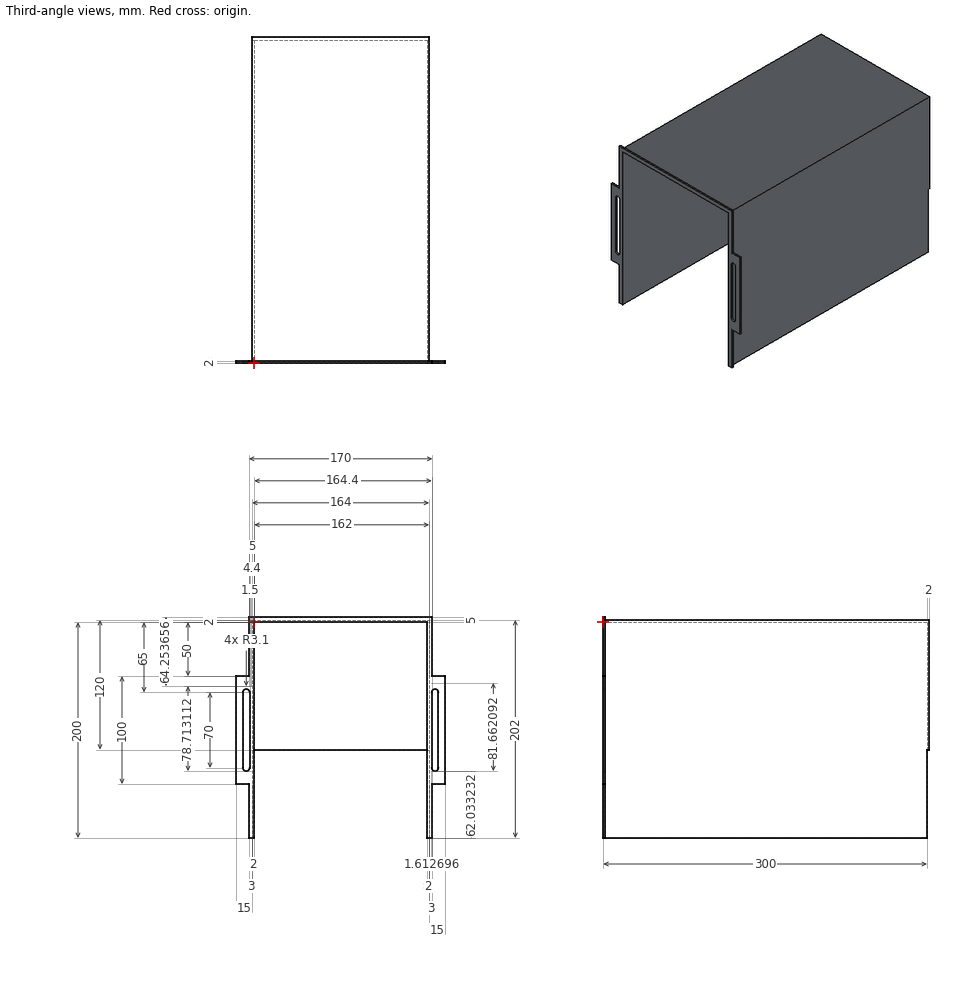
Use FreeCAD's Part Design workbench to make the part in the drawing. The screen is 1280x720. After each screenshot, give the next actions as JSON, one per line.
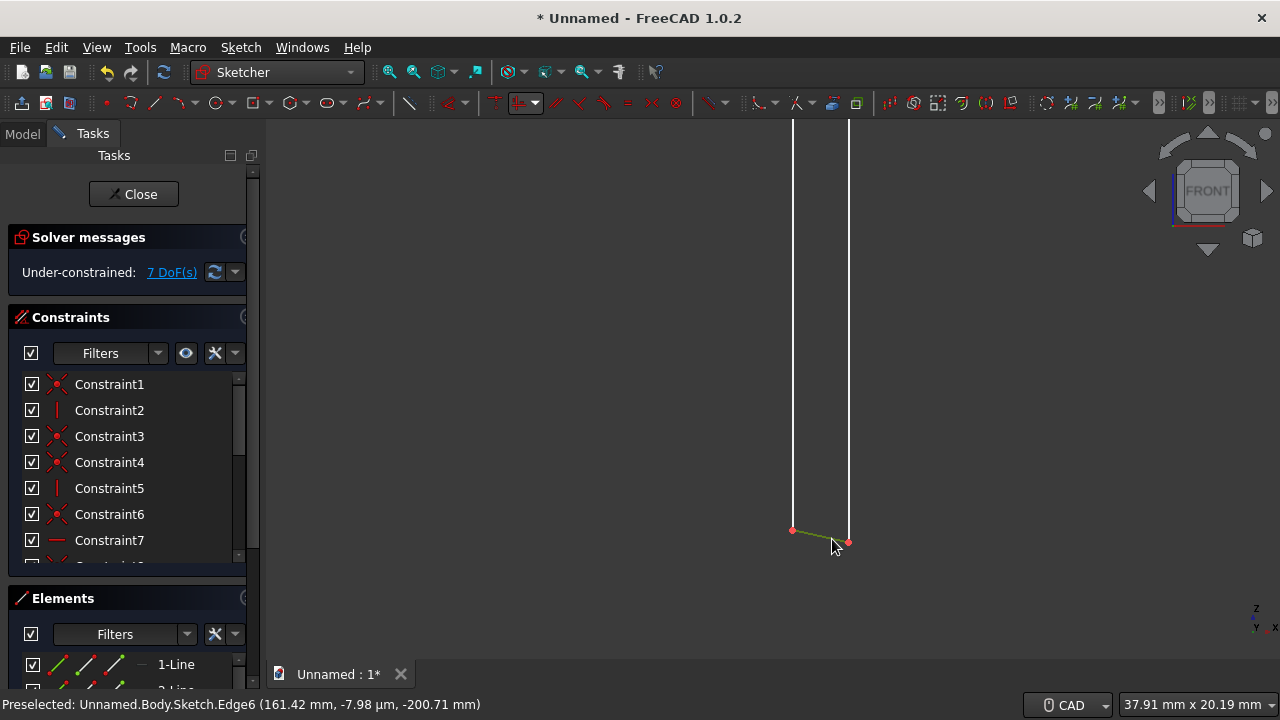
{"action": "key", "text": "h"}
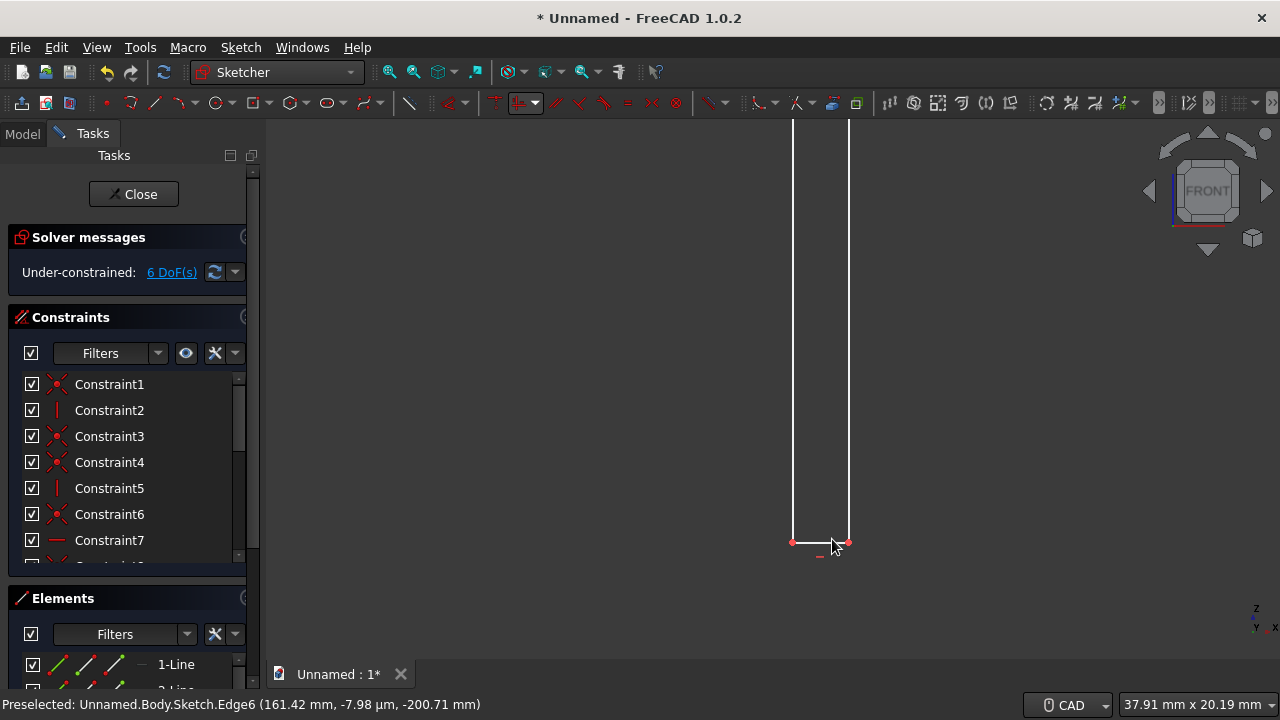
{"action": "left_click", "coordinate": [448, 104]}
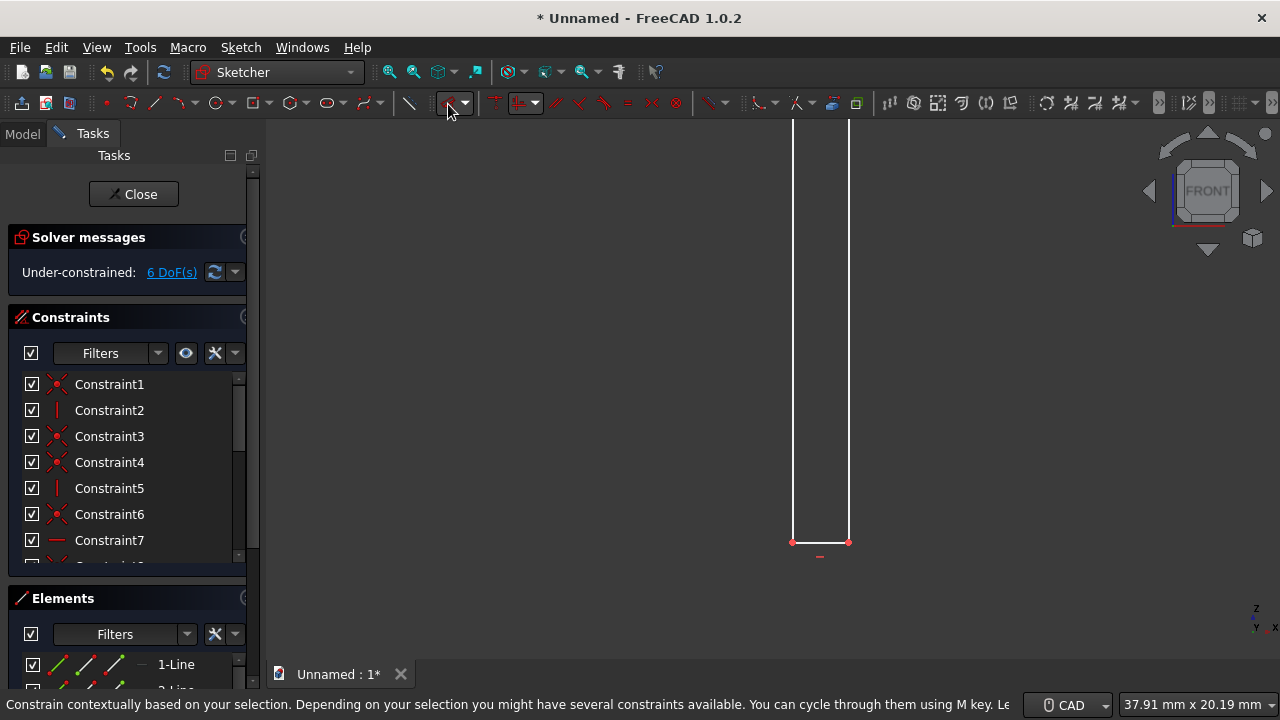
{"action": "scroll", "coordinate": [837, 555], "scroll_direction": "down", "scroll_amount": 14}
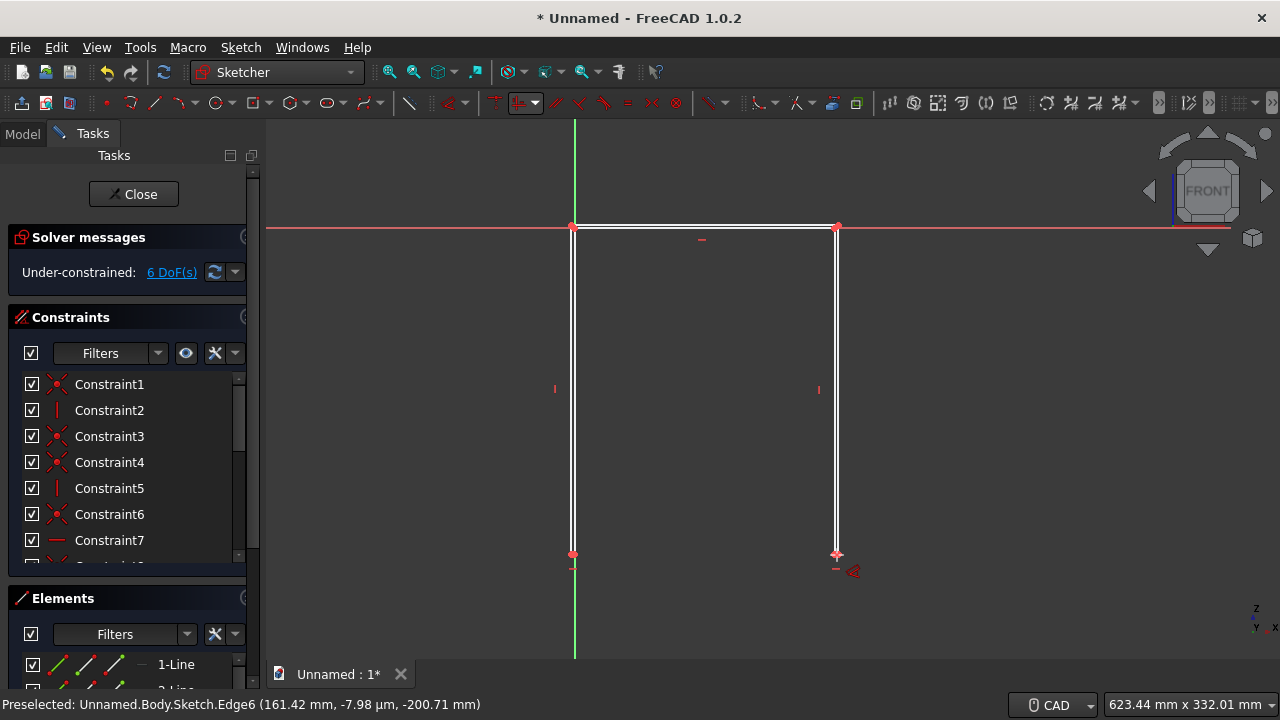
{"action": "scroll", "coordinate": [574, 555], "scroll_direction": "up", "scroll_amount": 14}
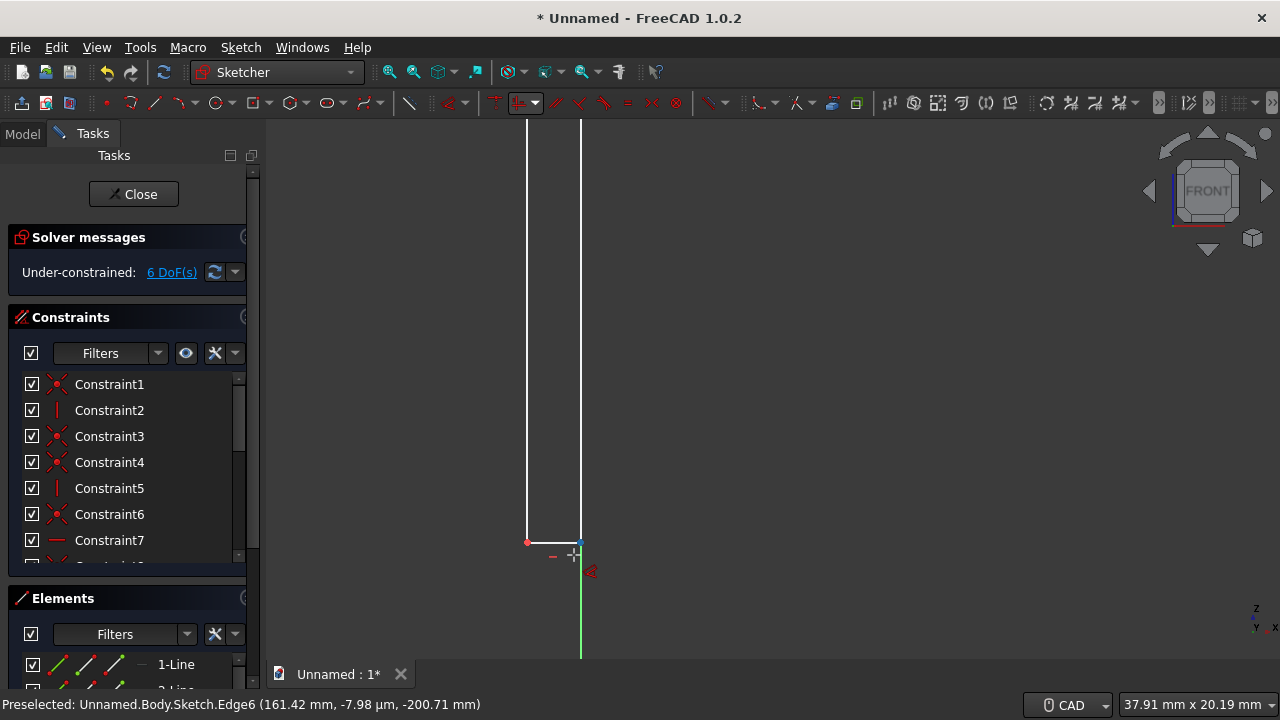
{"action": "left_click", "coordinate": [565, 543]}
{"action": "left_click", "coordinate": [554, 577]}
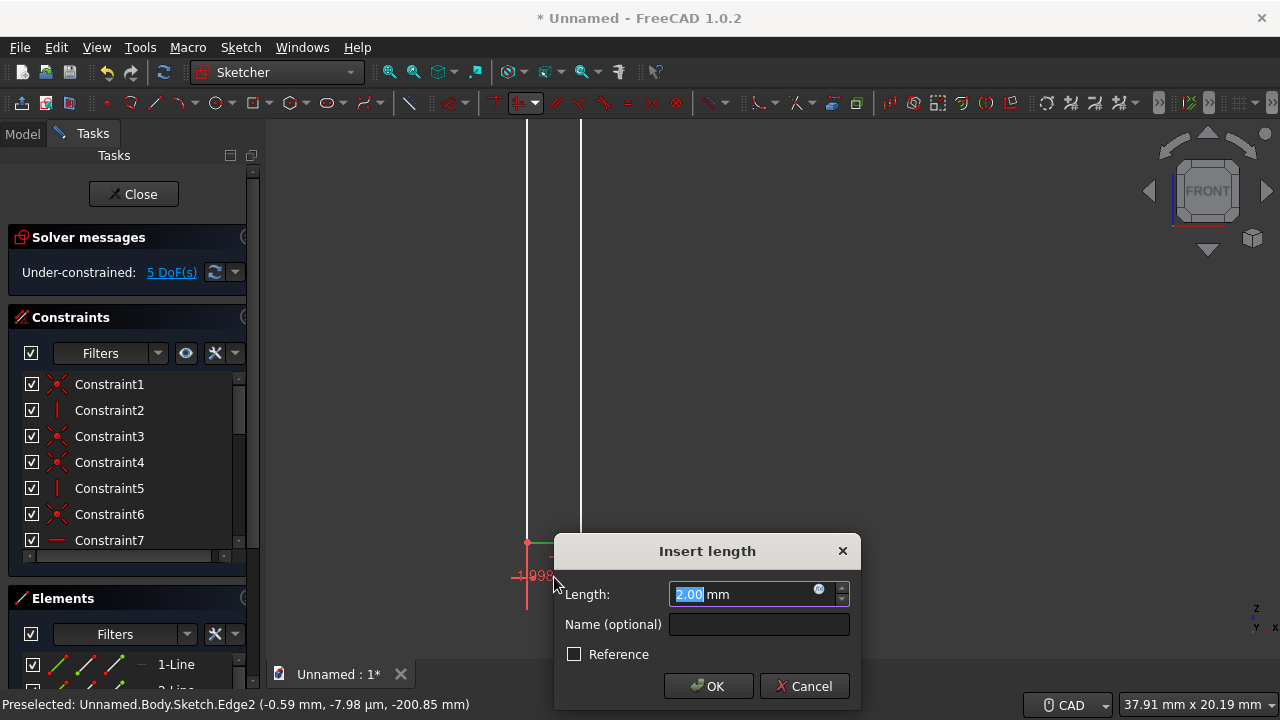
{"action": "type", "text": "2"}
{"action": "key", "text": "Return"}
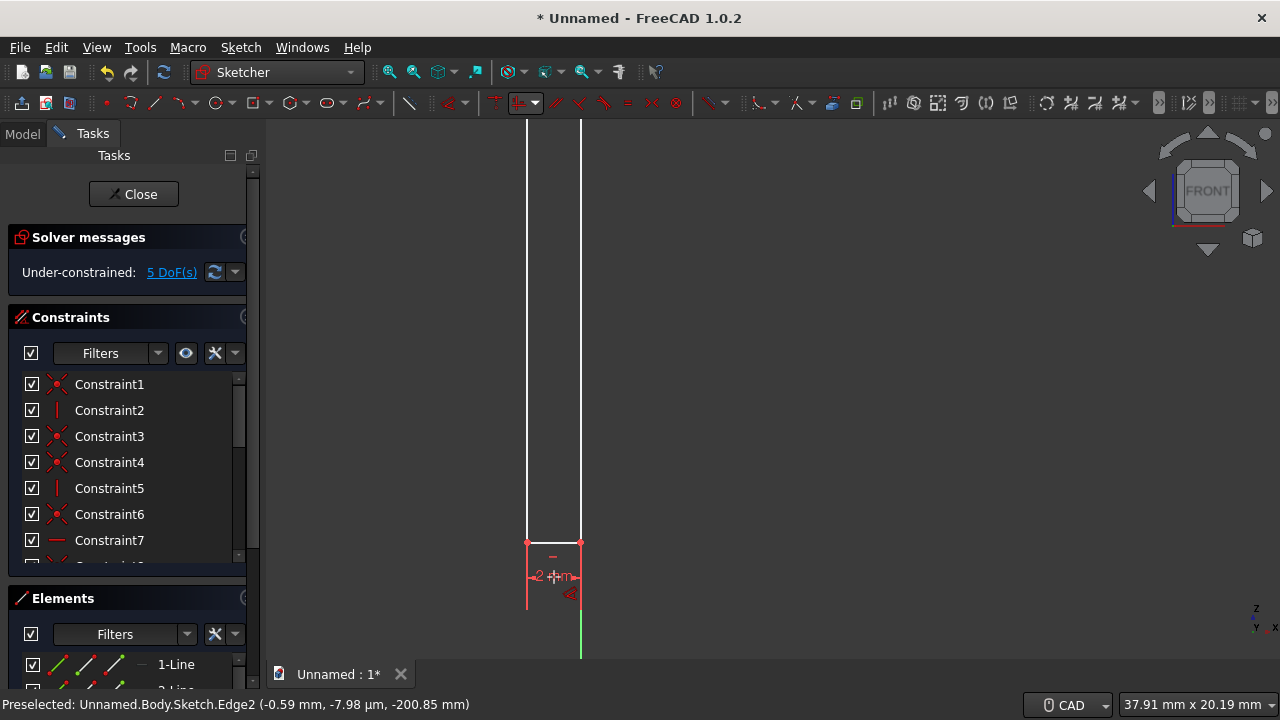
{"action": "scroll", "coordinate": [574, 555], "scroll_direction": "down", "scroll_amount": 14}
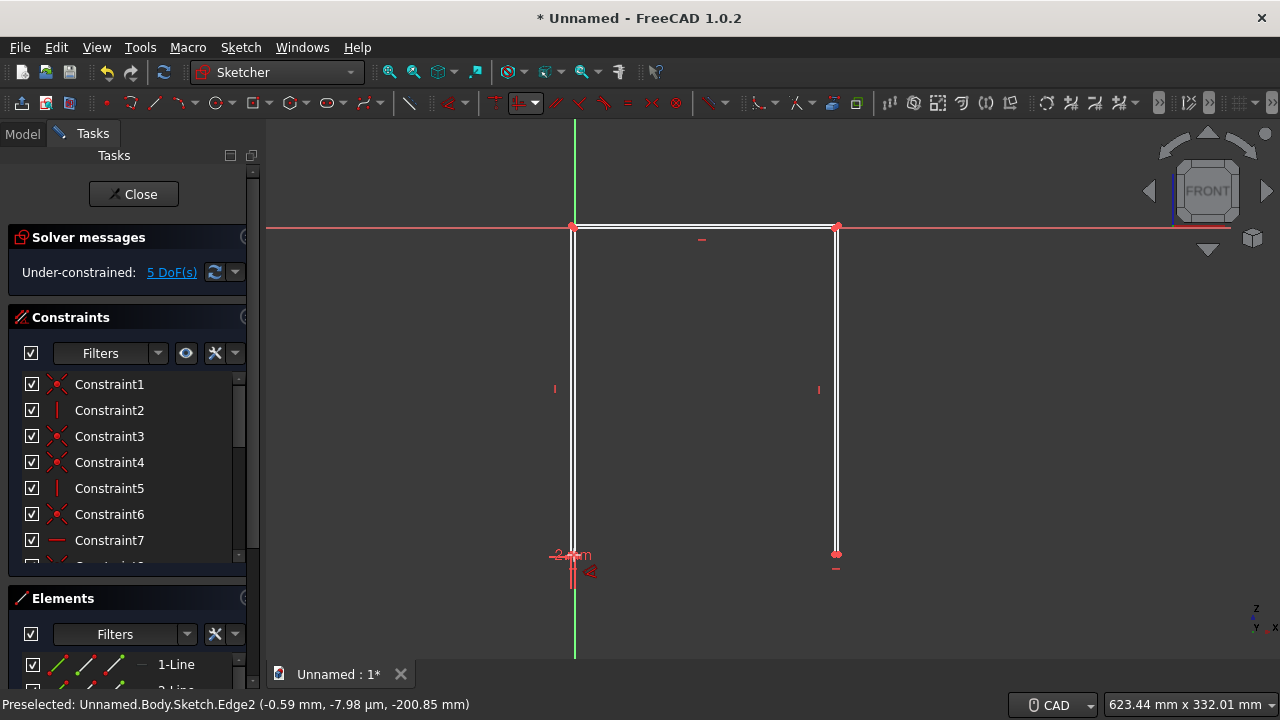
{"action": "scroll", "coordinate": [837, 555], "scroll_direction": "up", "scroll_amount": 14}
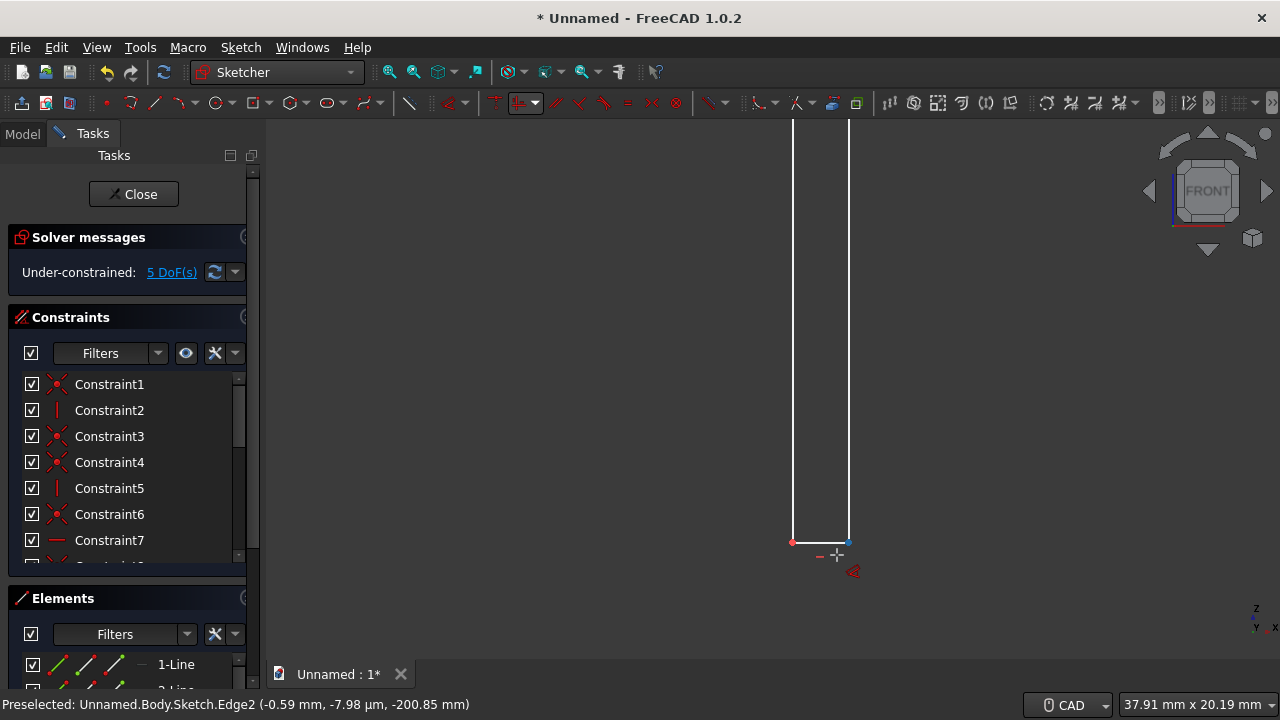
{"action": "left_click", "coordinate": [832, 543]}
{"action": "left_click", "coordinate": [821, 577]}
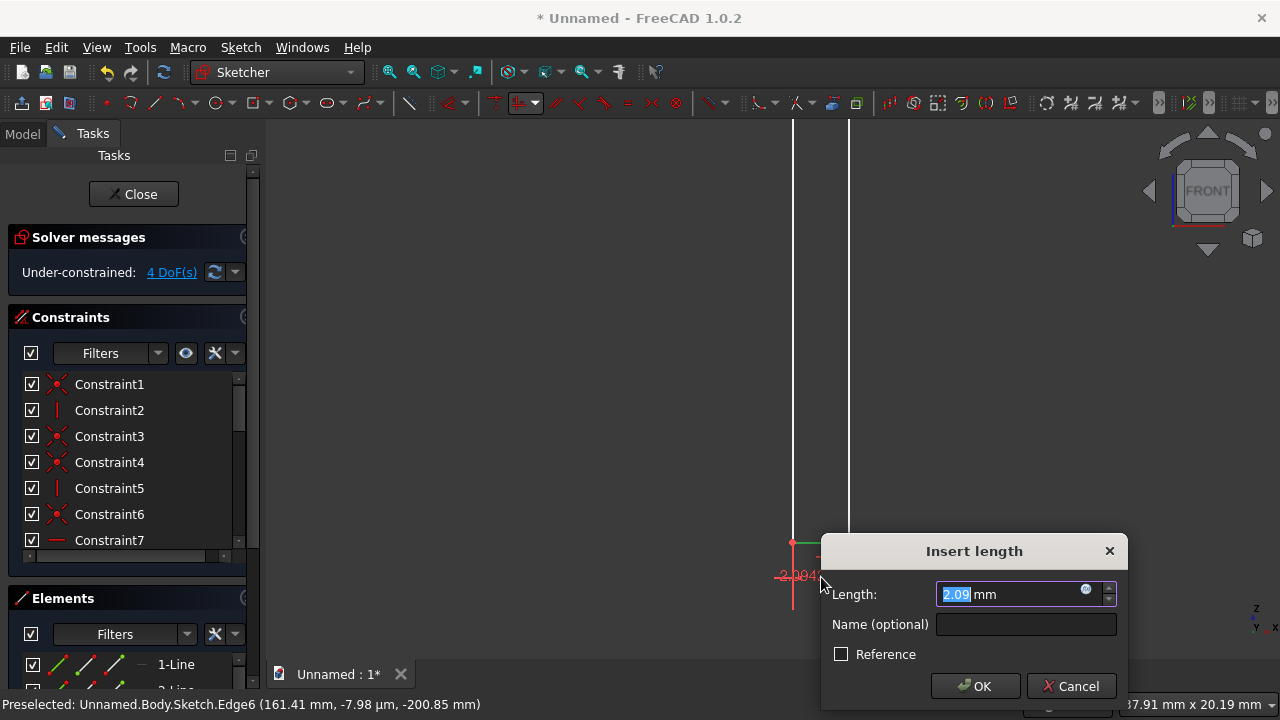
{"action": "type", "text": "2"}
{"action": "key", "text": "Return"}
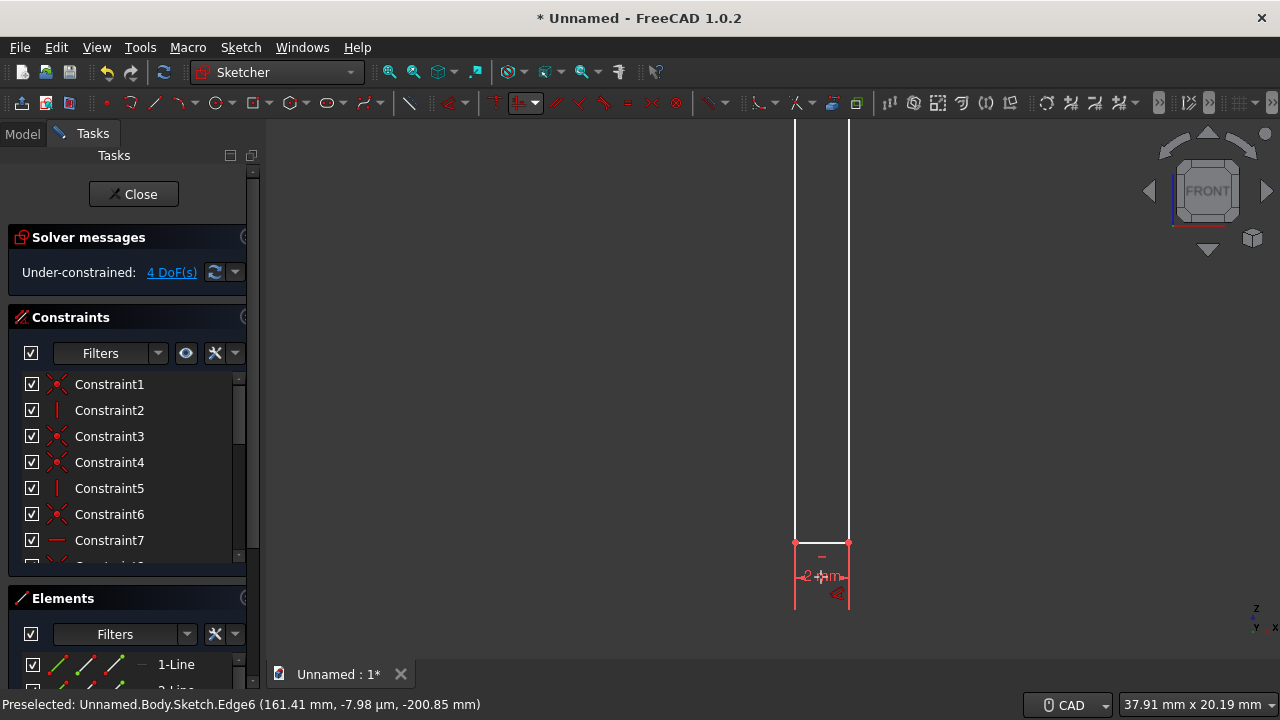
{"action": "scroll", "coordinate": [837, 555], "scroll_direction": "down", "scroll_amount": 14}